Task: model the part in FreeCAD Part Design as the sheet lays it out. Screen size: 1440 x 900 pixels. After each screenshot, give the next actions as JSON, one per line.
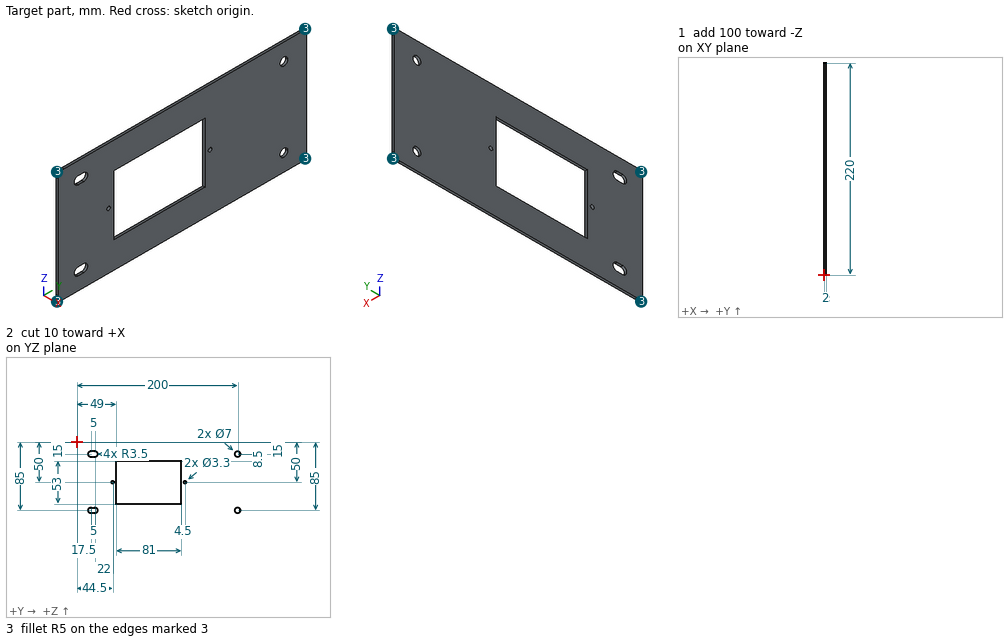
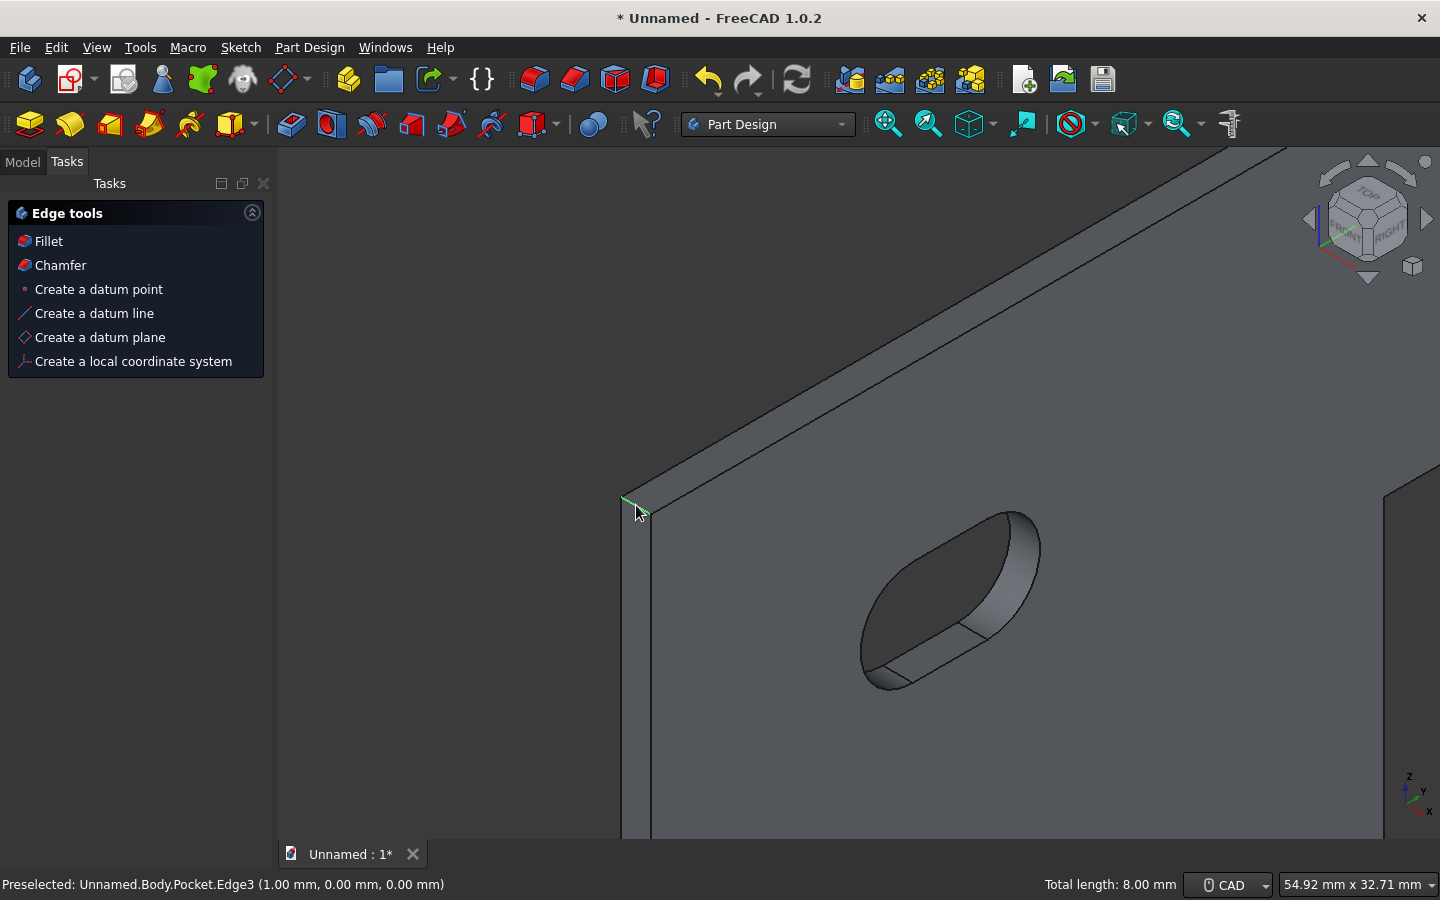
{"action": "left_click", "coordinate": [536, 80]}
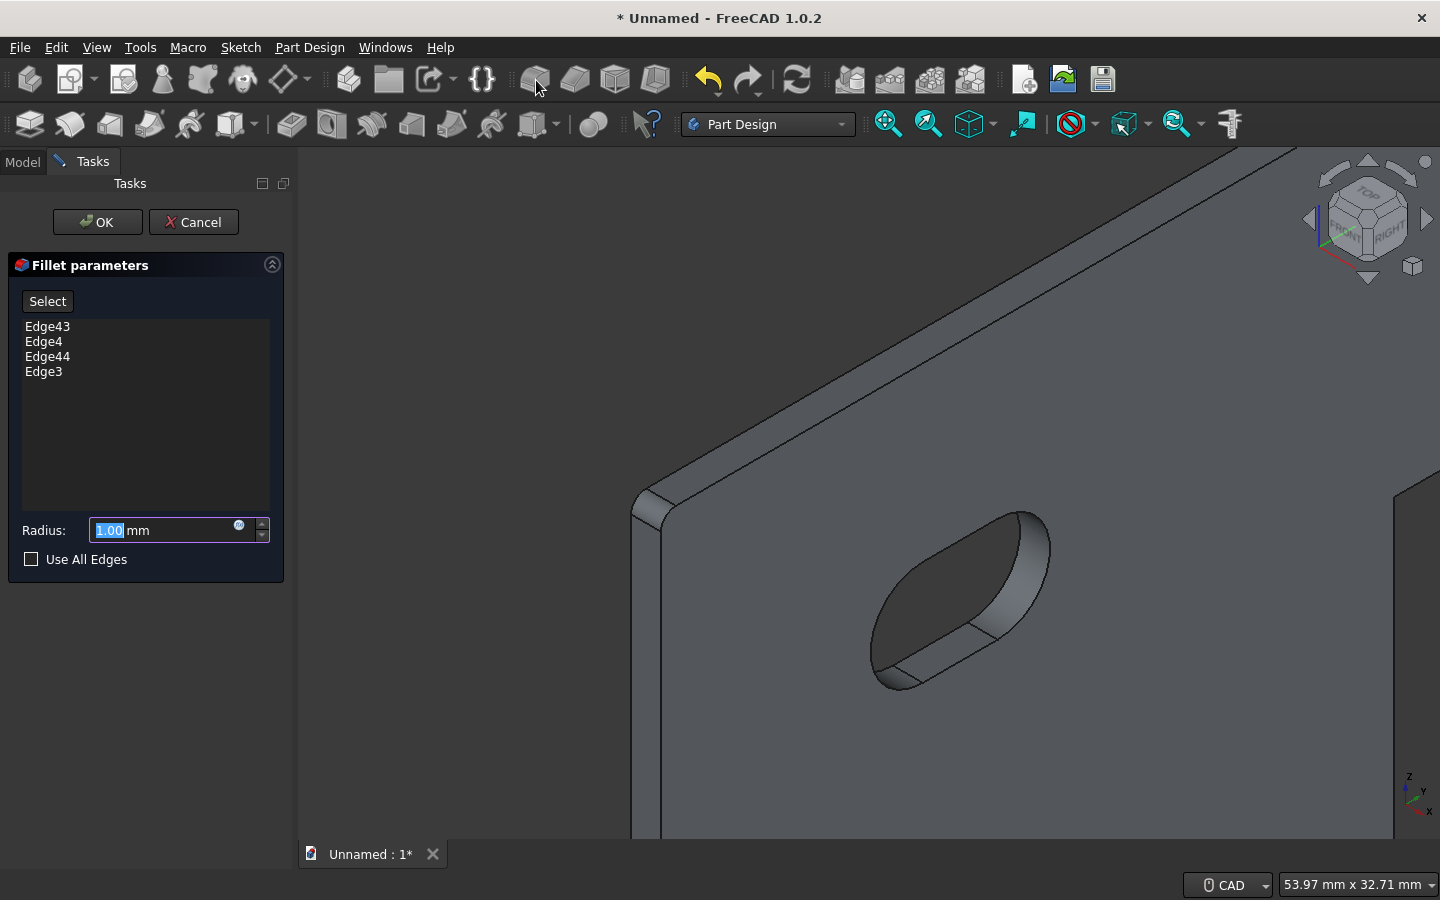
{"action": "type", "text": "5"}
{"action": "key", "text": "Tab"}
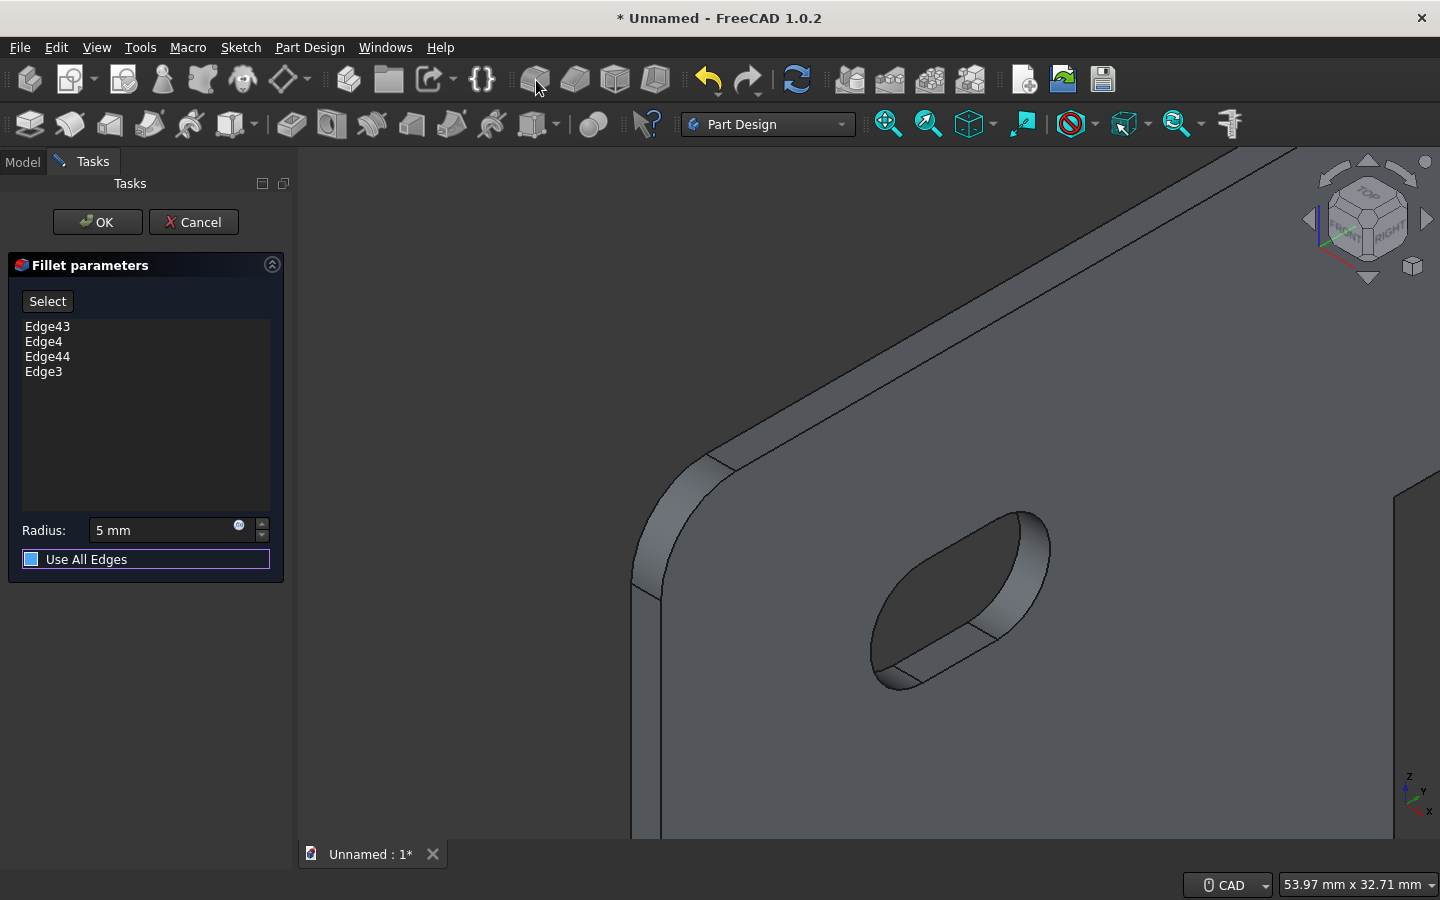
{"action": "left_click", "coordinate": [98, 222]}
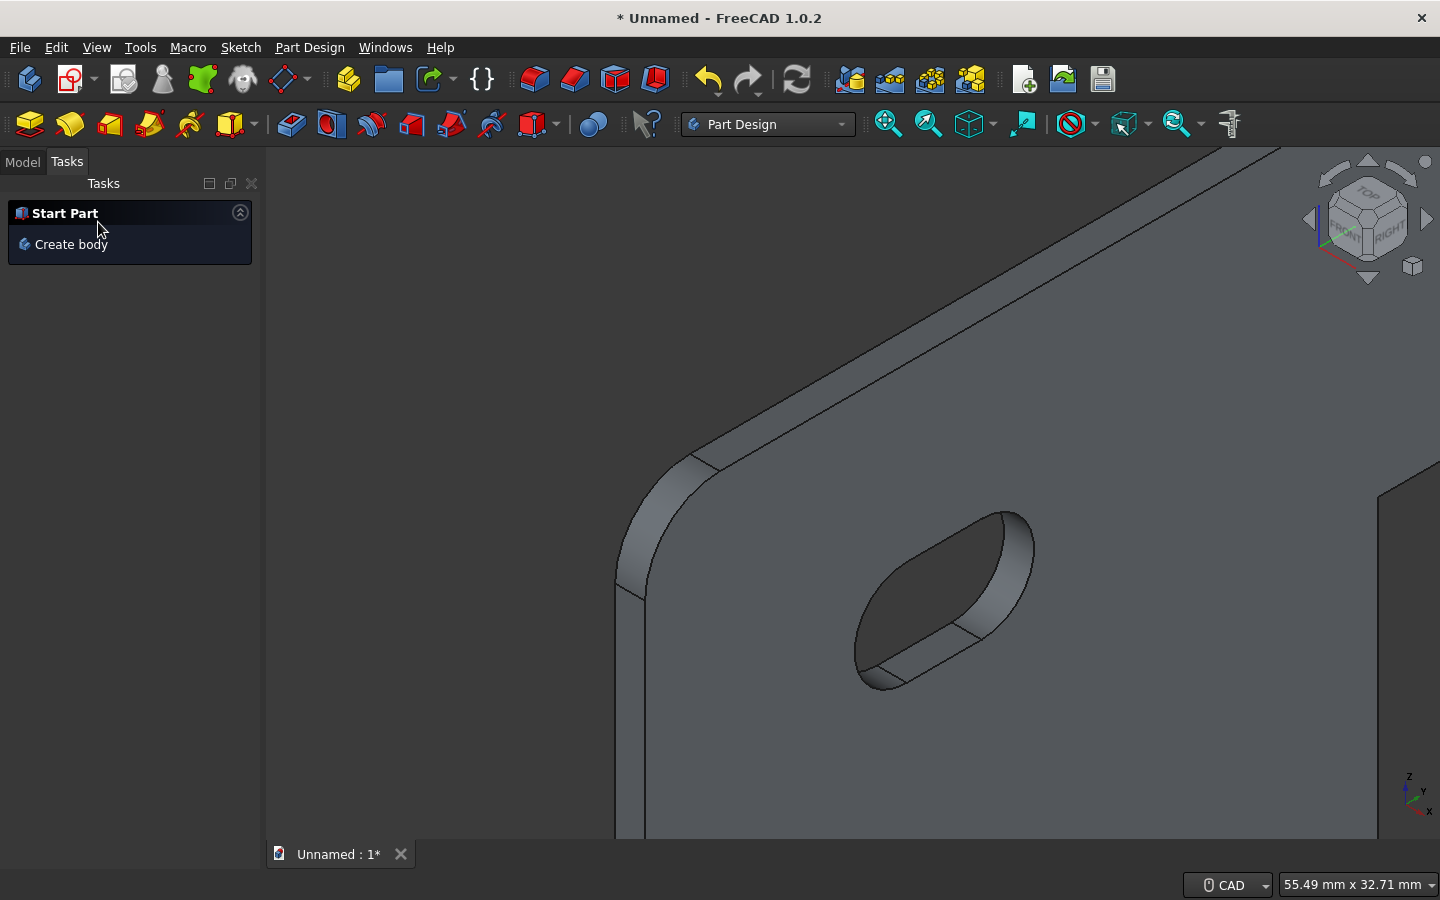
{"action": "left_click", "coordinate": [890, 124]}